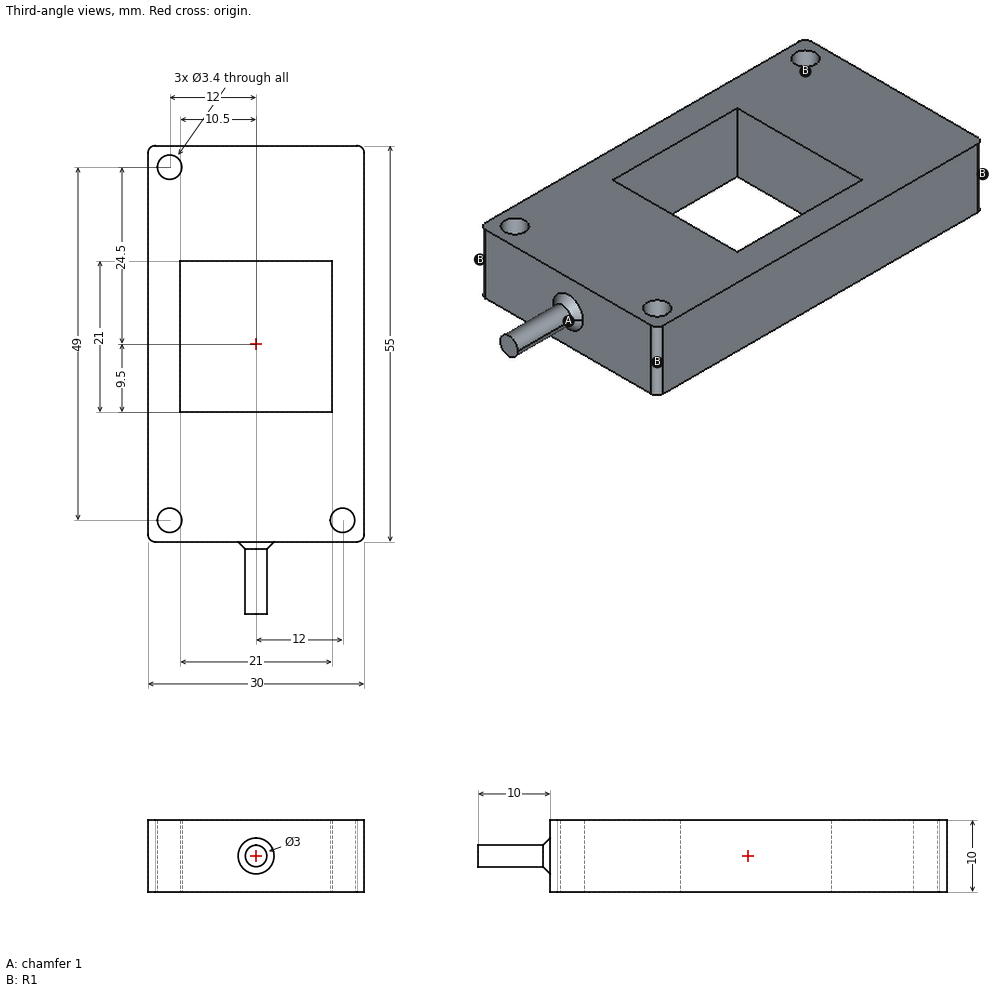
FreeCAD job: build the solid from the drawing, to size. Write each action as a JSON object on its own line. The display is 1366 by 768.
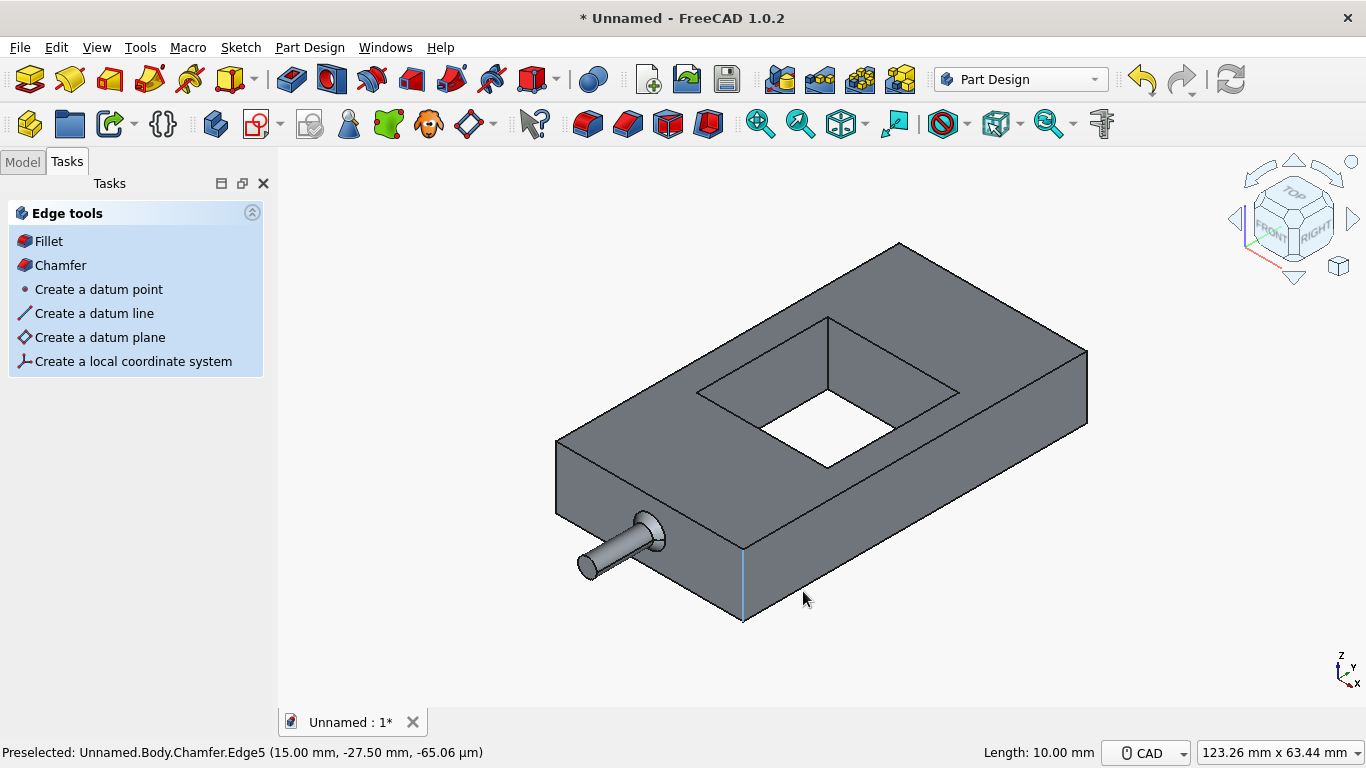
{"action": "key", "text": "2"}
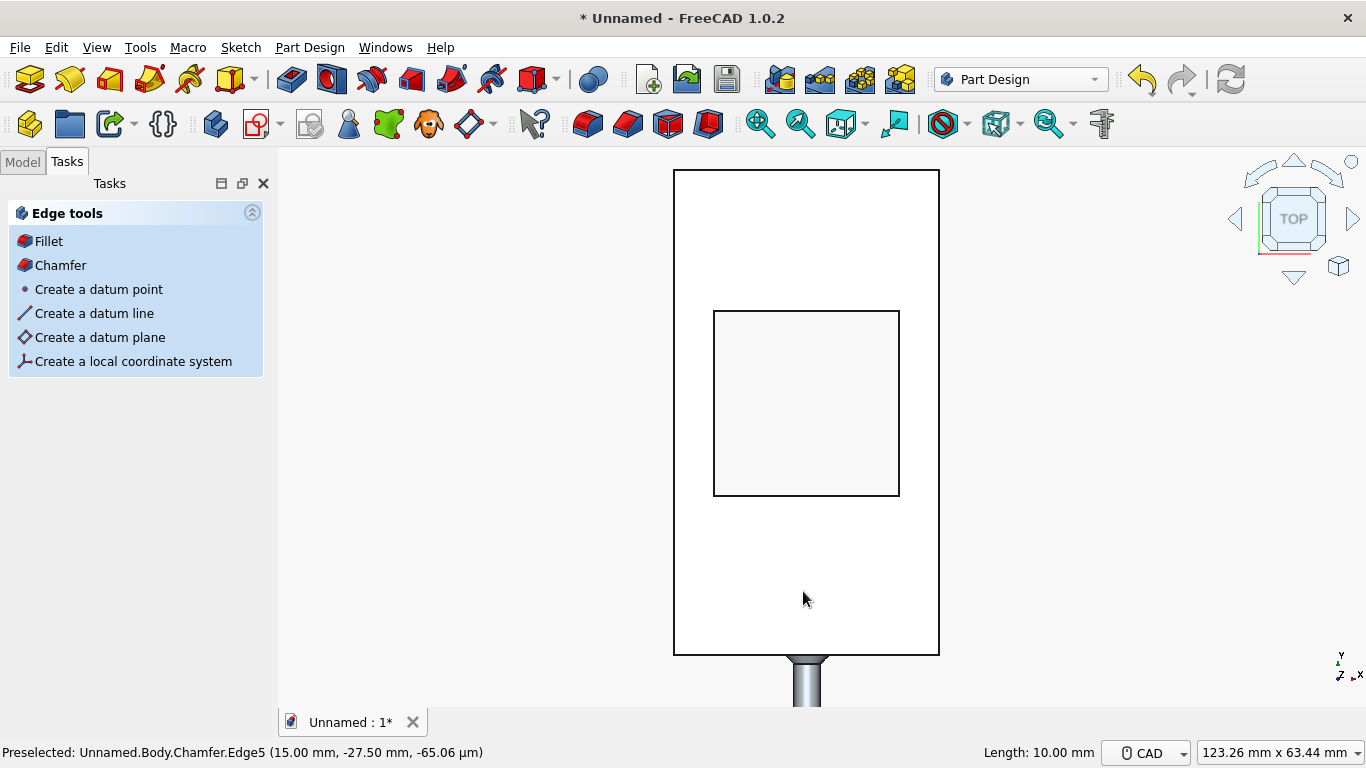
{"action": "left_click", "coordinate": [762, 124]}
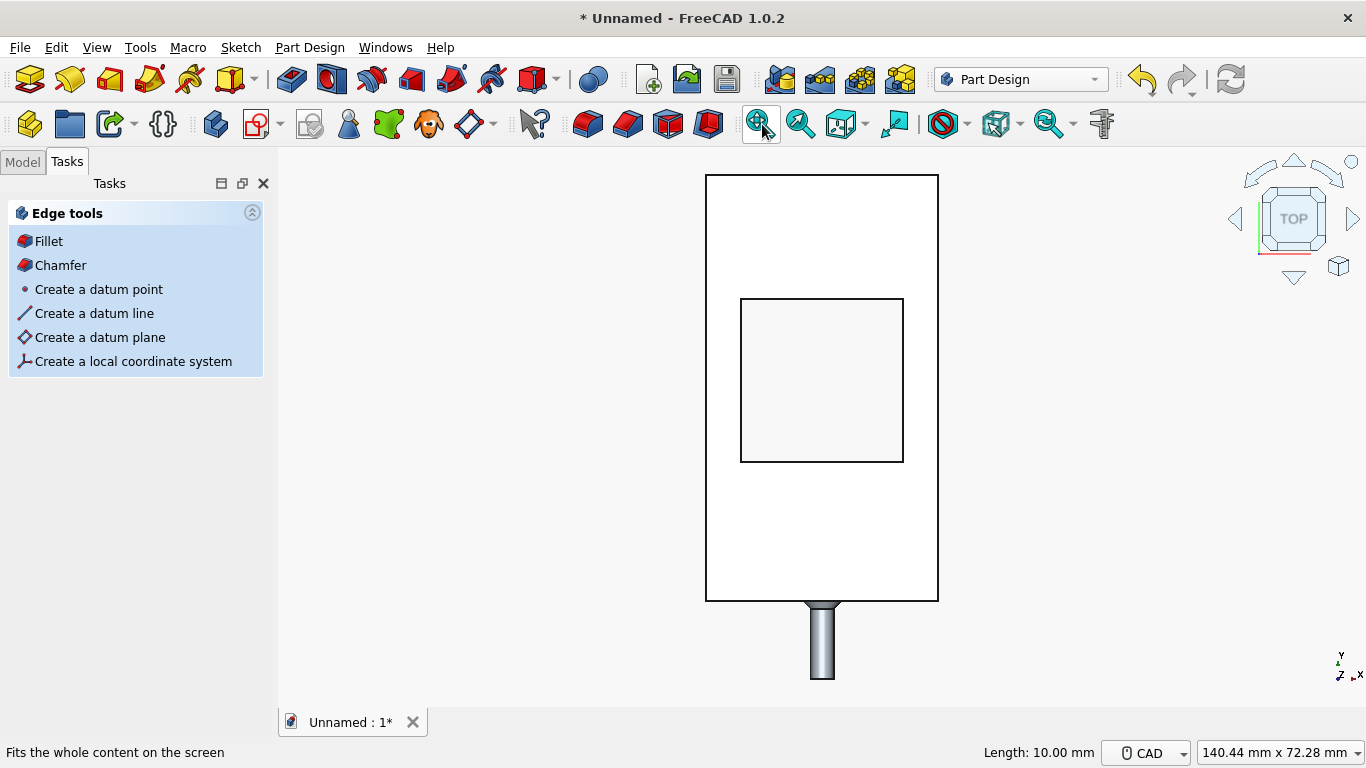
{"action": "key", "text": "1"}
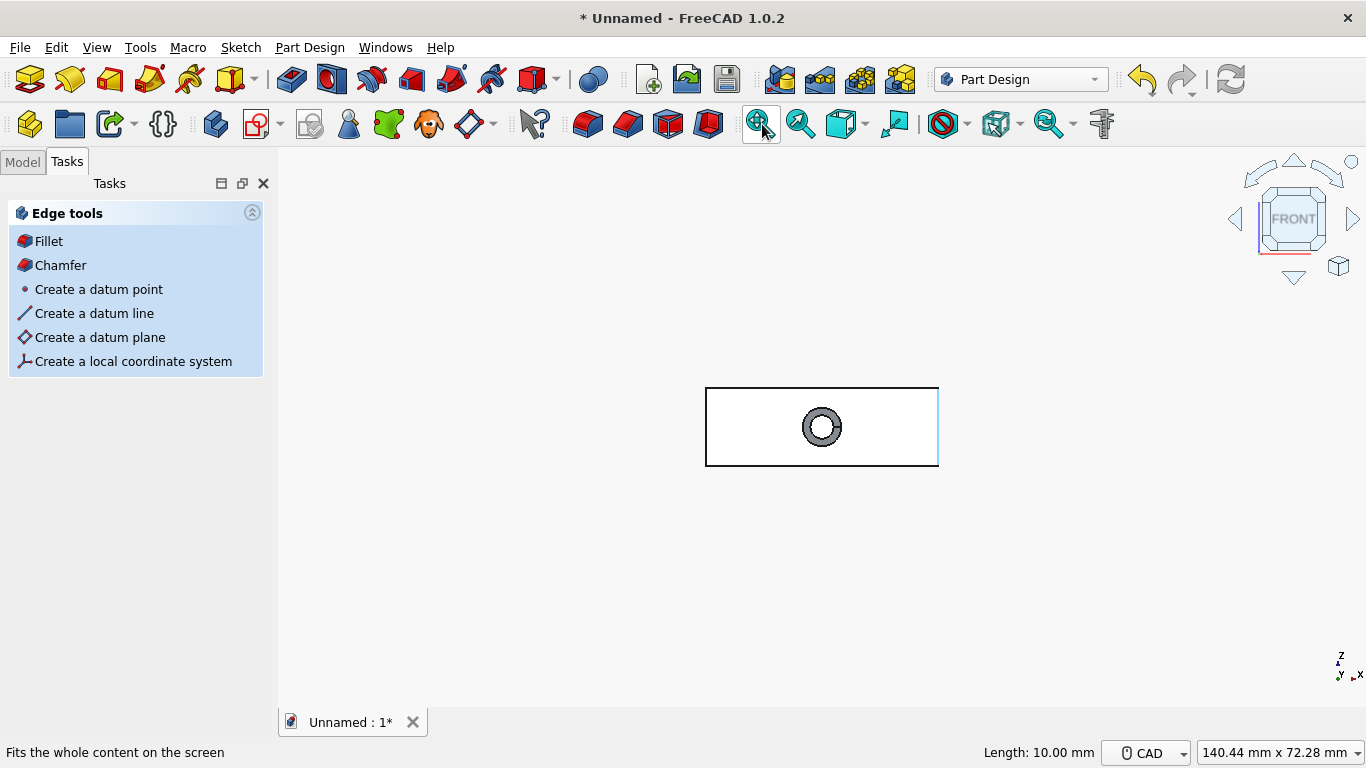
{"action": "key", "text": "v f"}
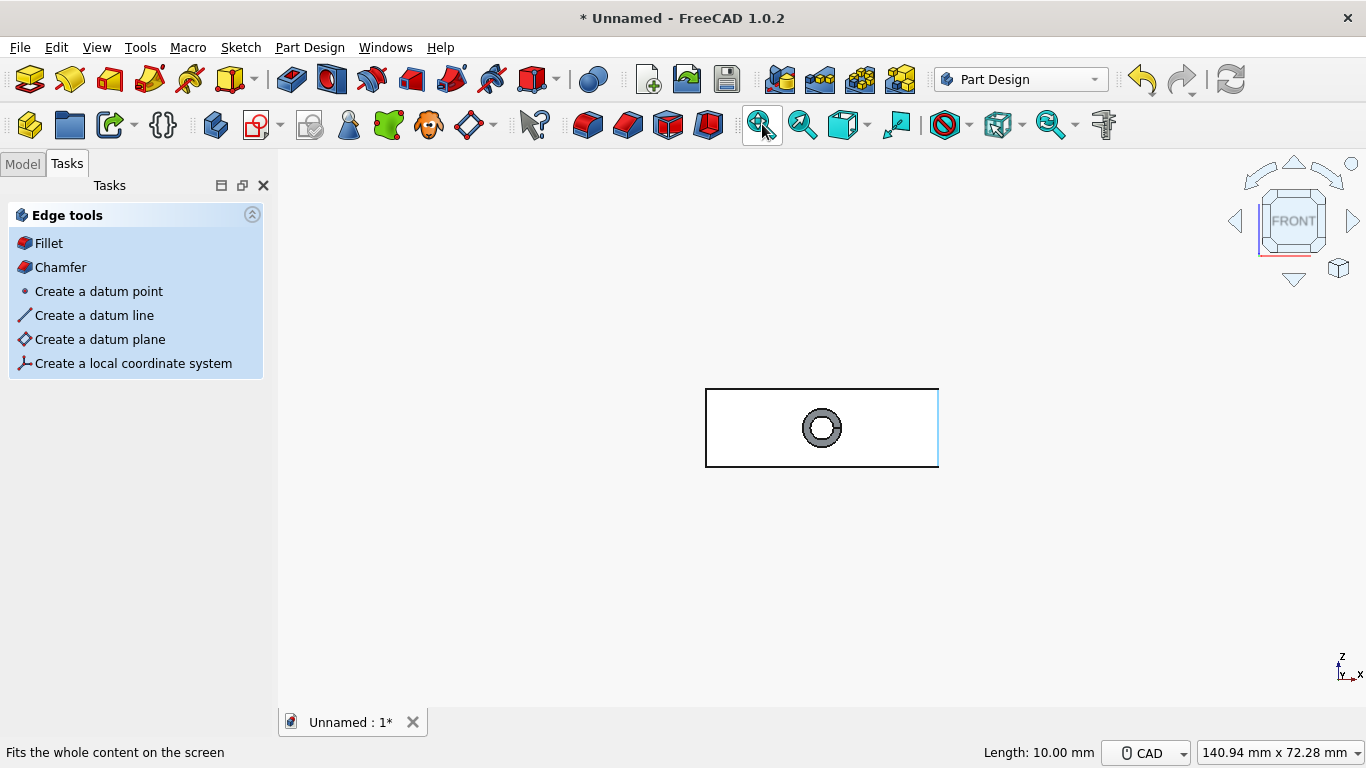
{"action": "left_click", "coordinate": [706, 427], "text": "ctrl"}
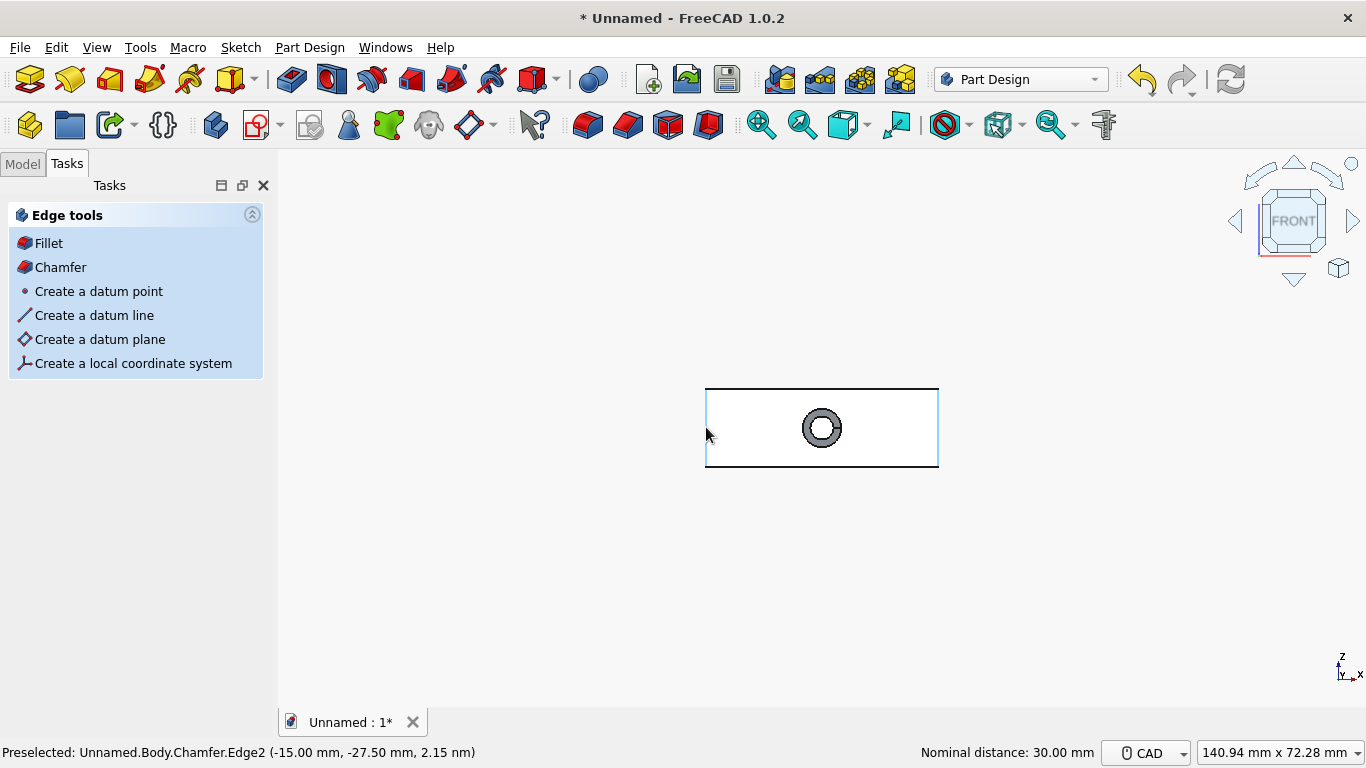
{"action": "key", "text": "3"}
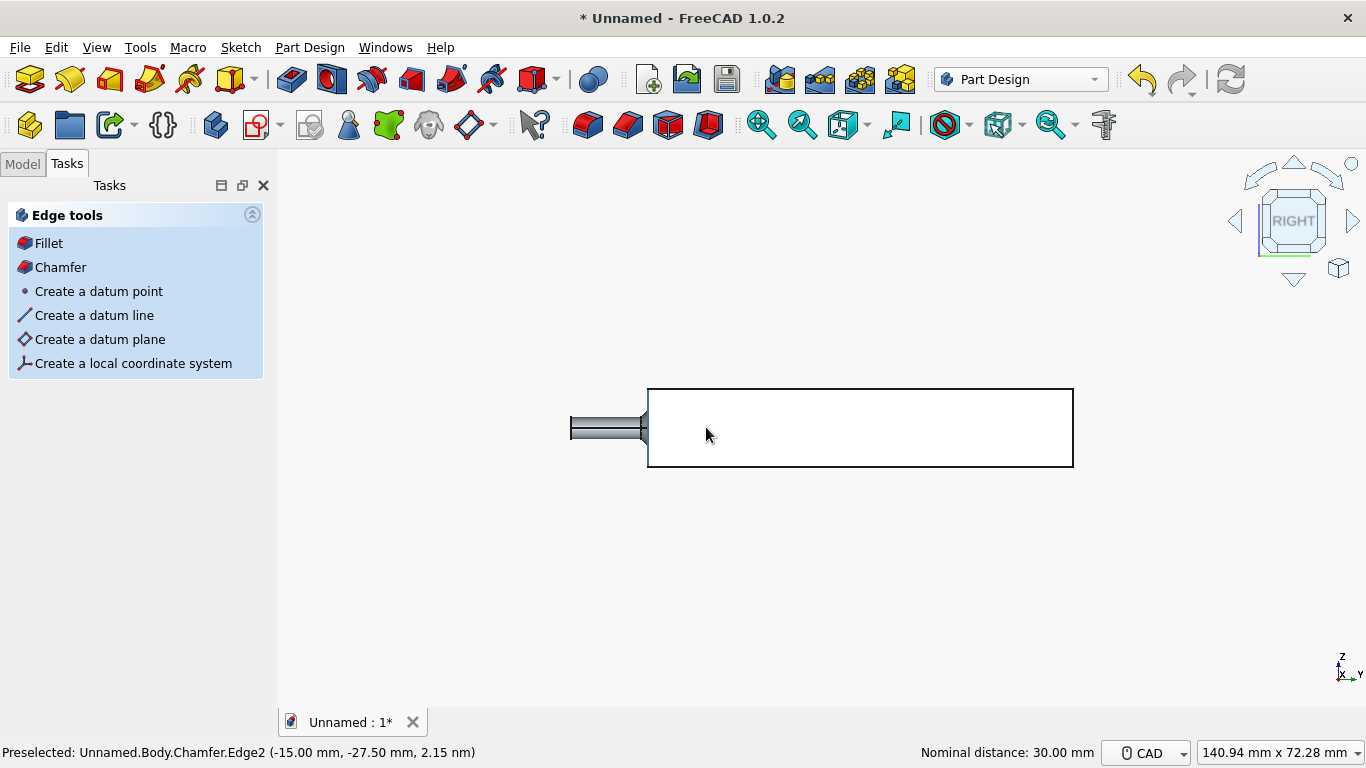
{"action": "left_click", "coordinate": [1073, 427], "text": "ctrl"}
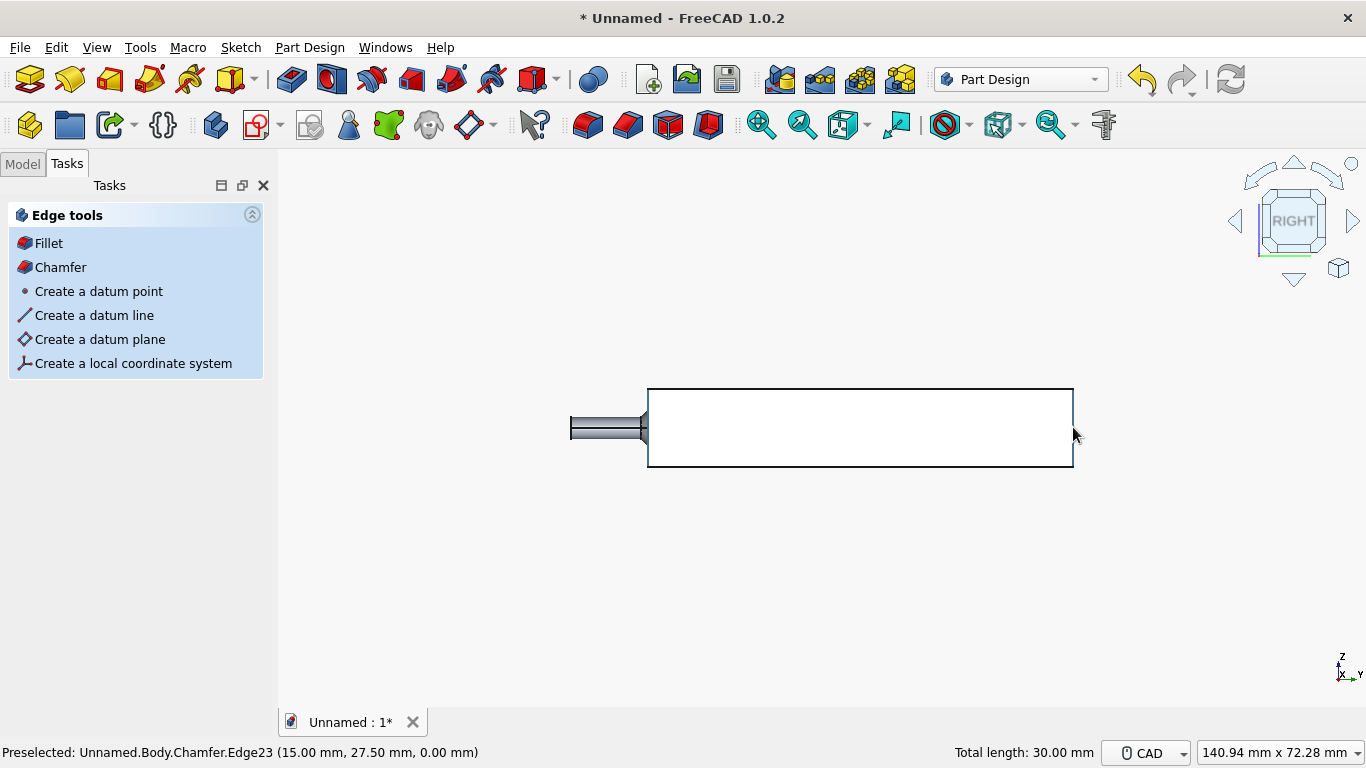
{"action": "key", "text": "5"}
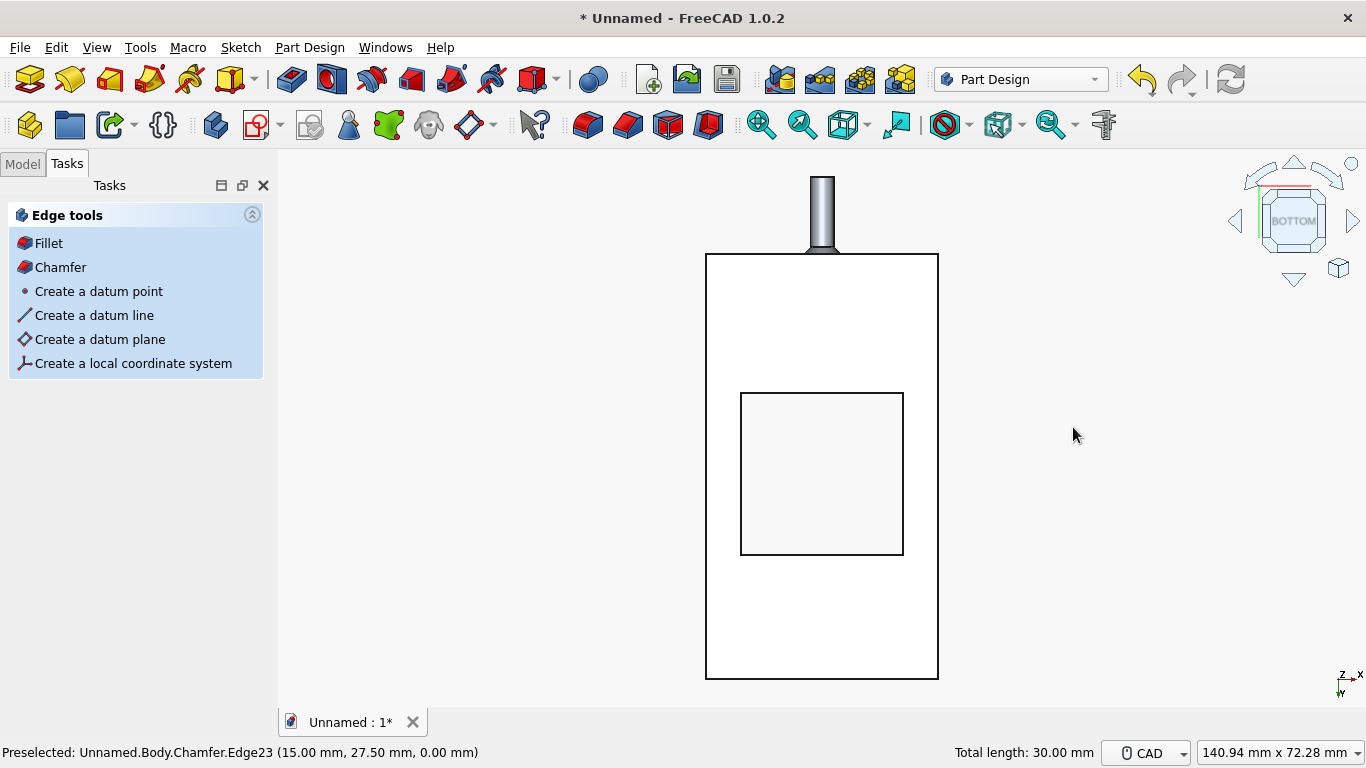
{"action": "key", "text": "4"}